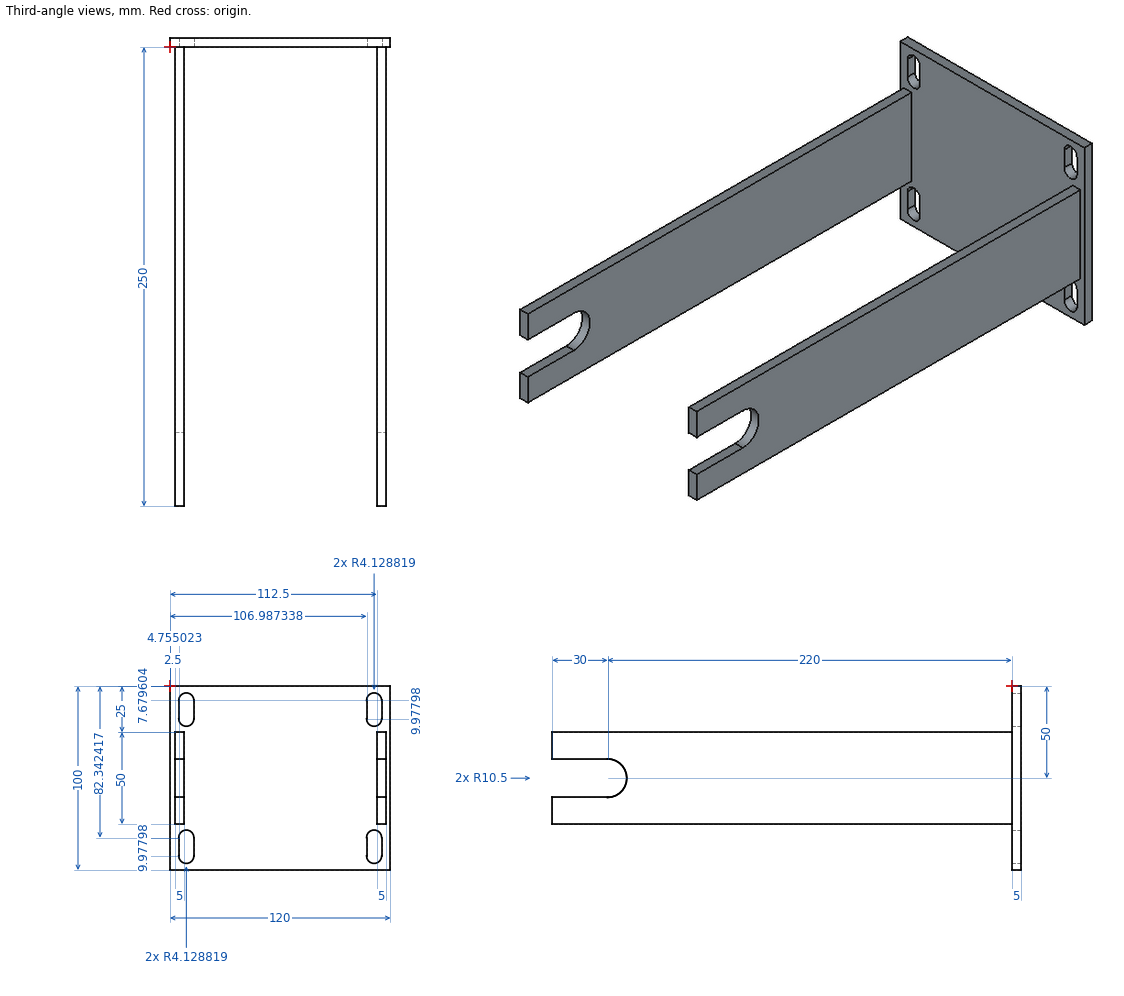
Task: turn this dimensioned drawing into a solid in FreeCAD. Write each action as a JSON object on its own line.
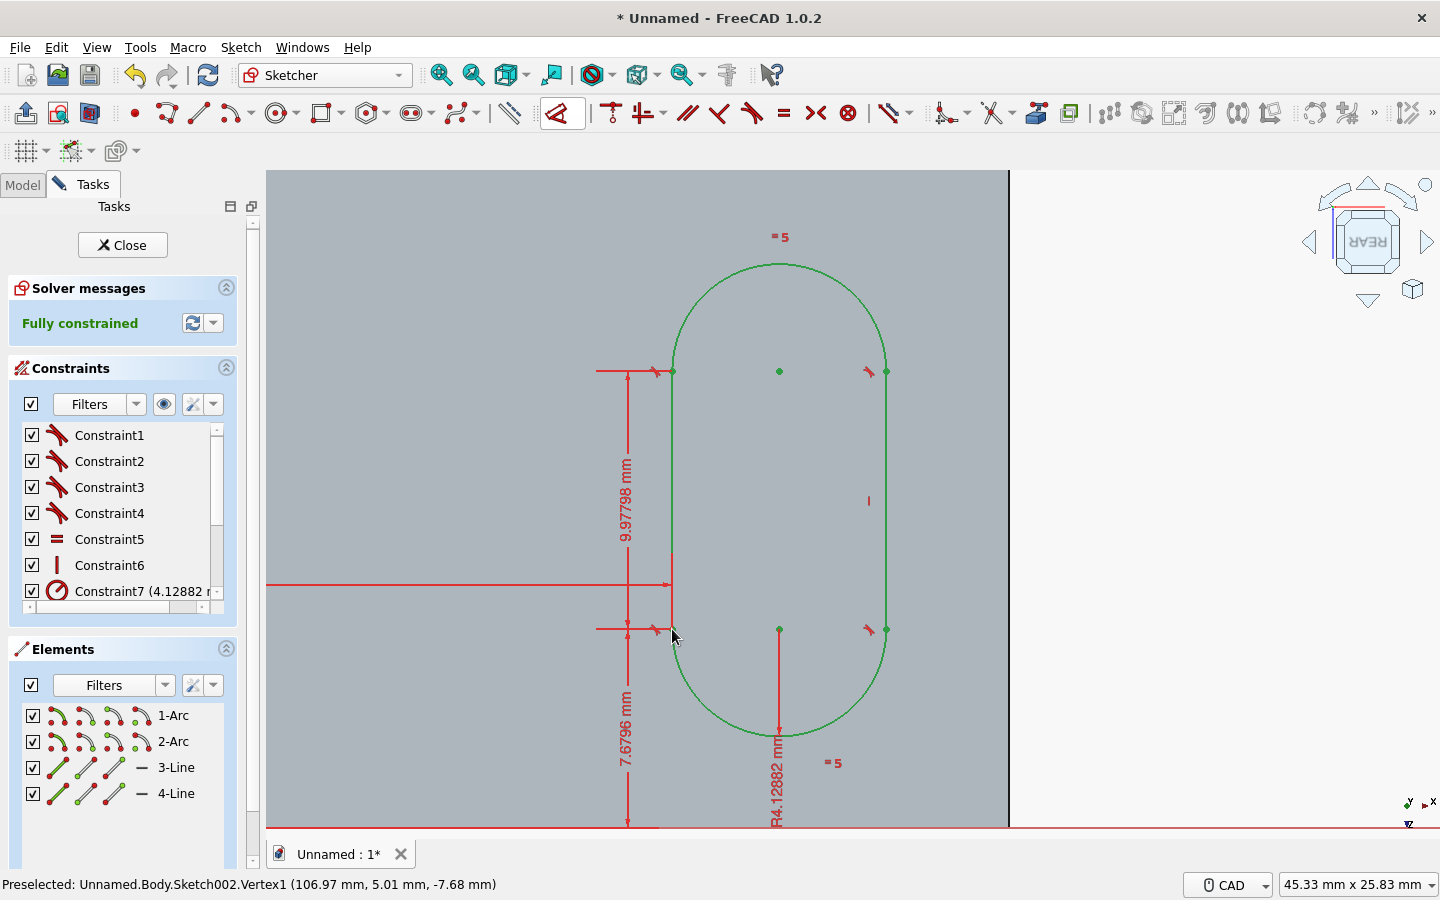
{"action": "left_click", "coordinate": [123, 245]}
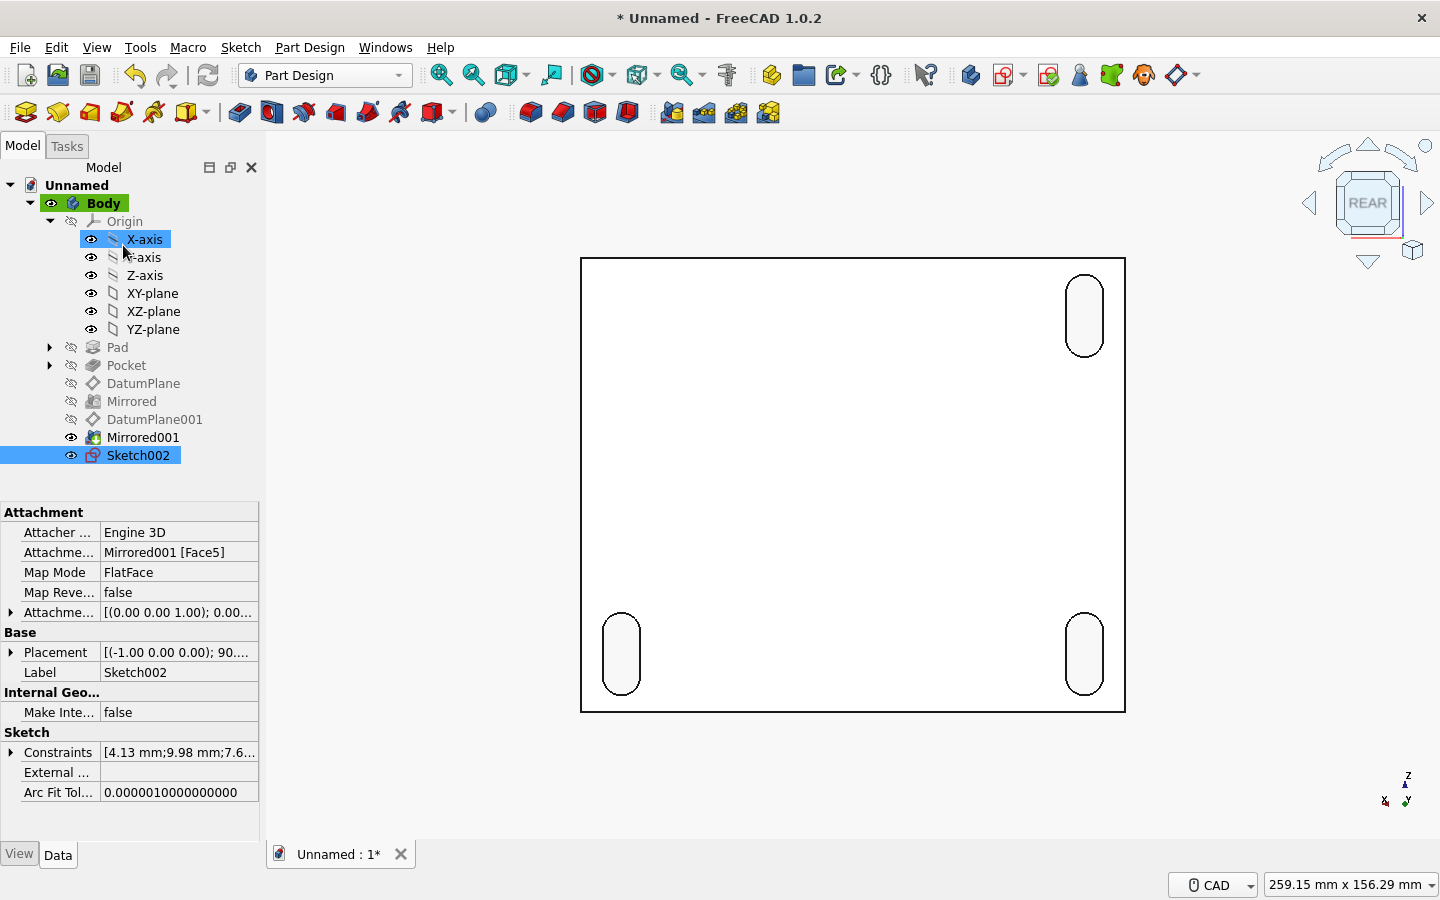
{"action": "left_click", "coordinate": [240, 112]}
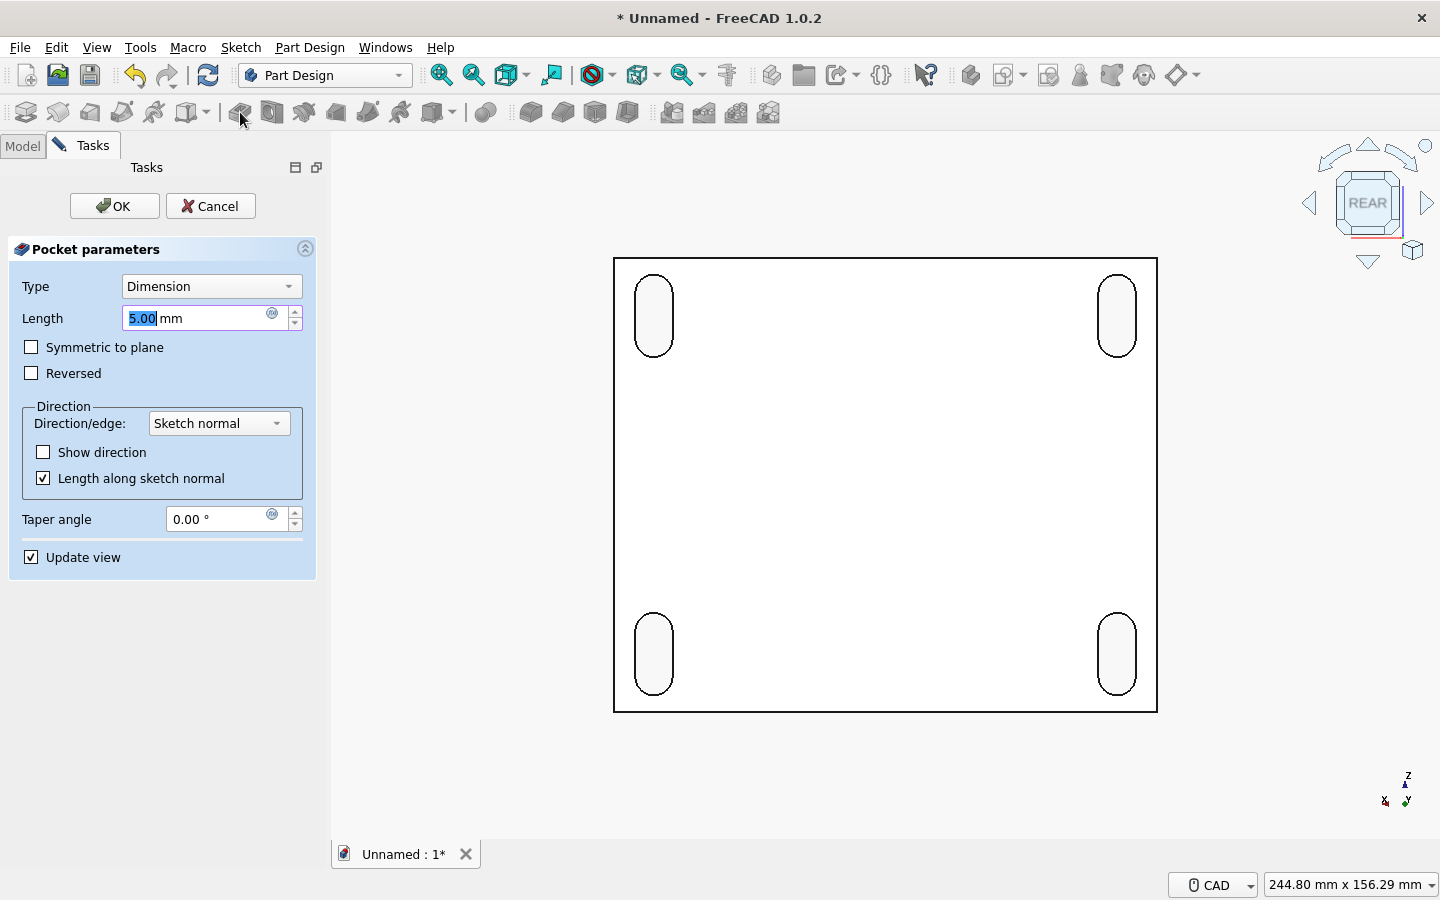
{"action": "left_click", "coordinate": [212, 286]}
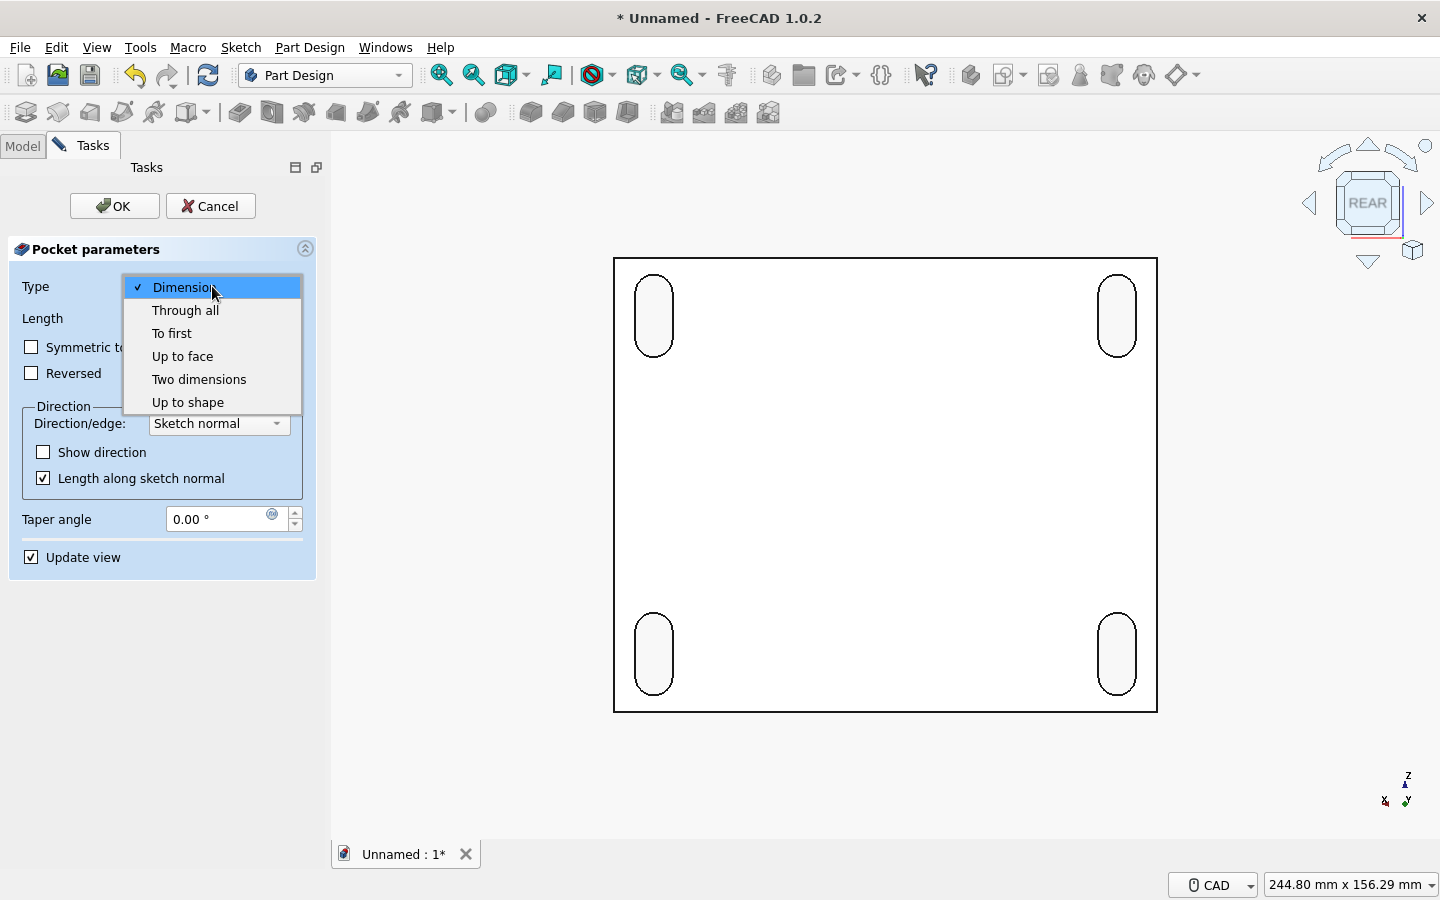
{"action": "left_click", "coordinate": [212, 310]}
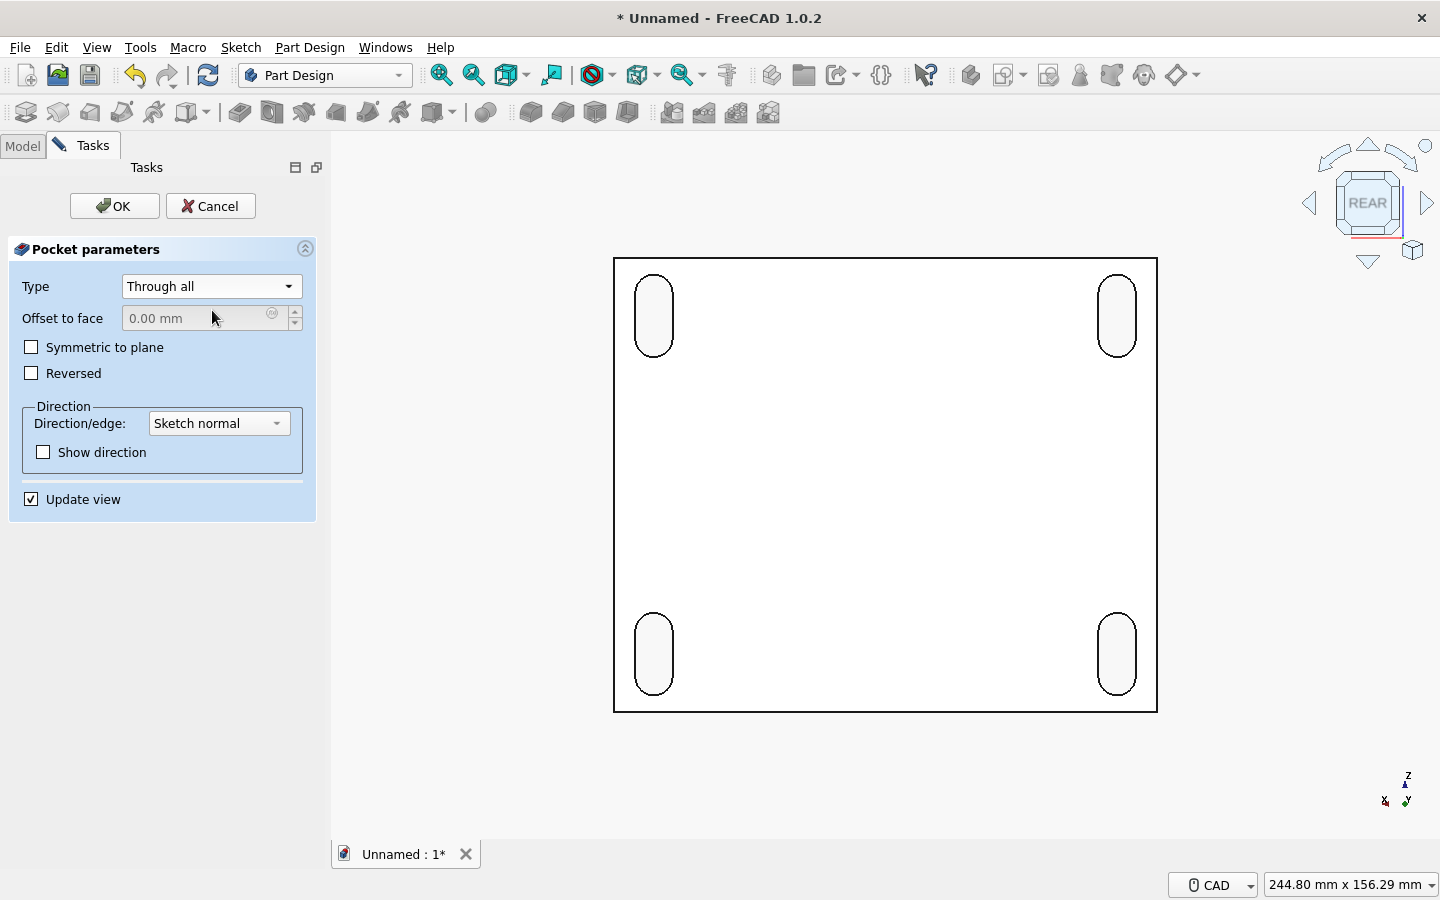
{"action": "left_click", "coordinate": [115, 206]}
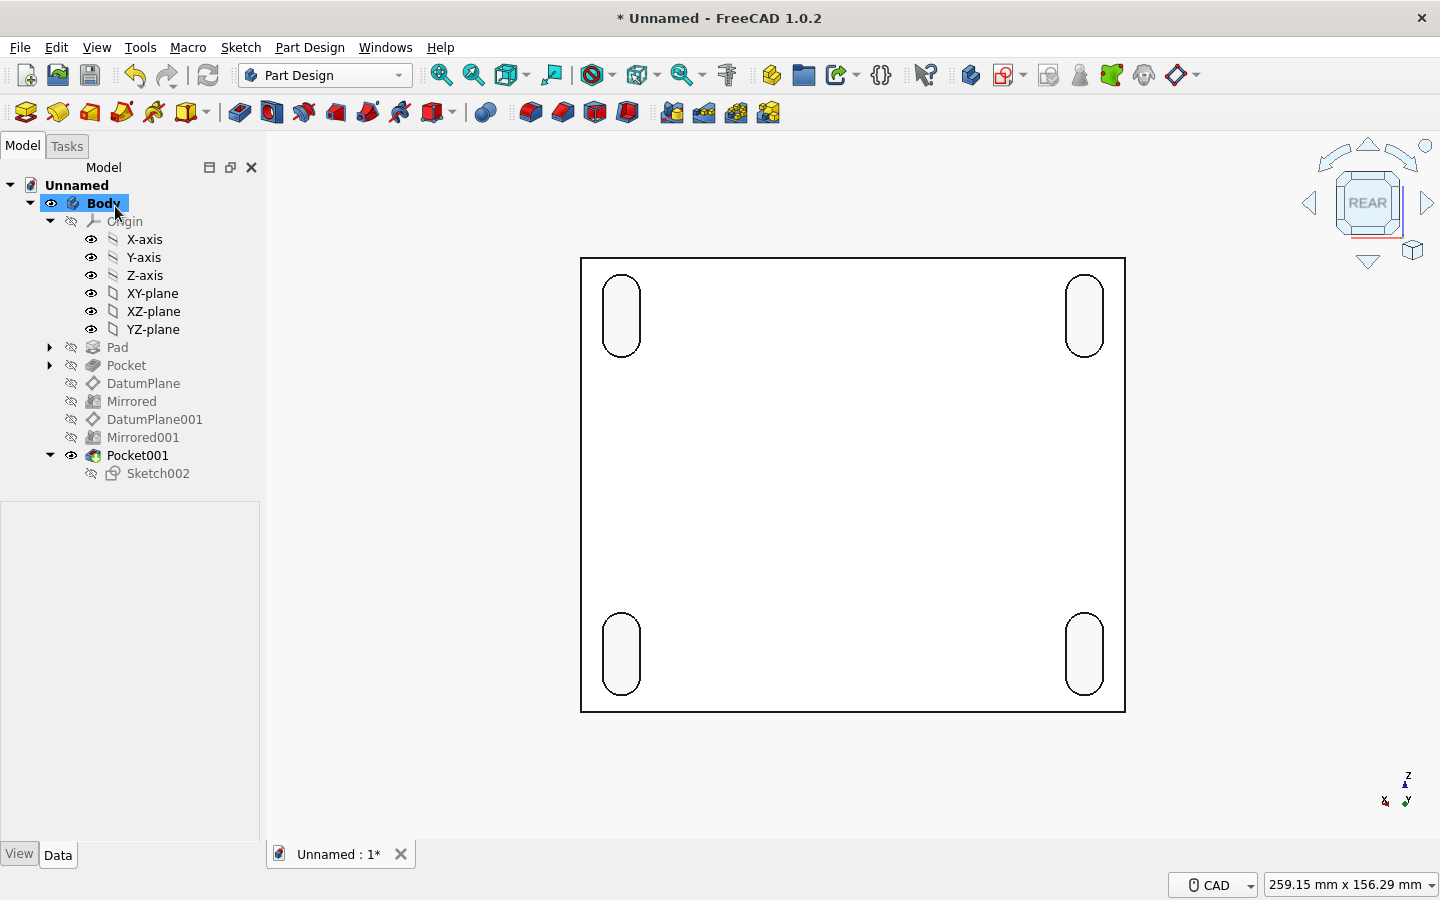
{"action": "left_click", "coordinate": [1004, 76]}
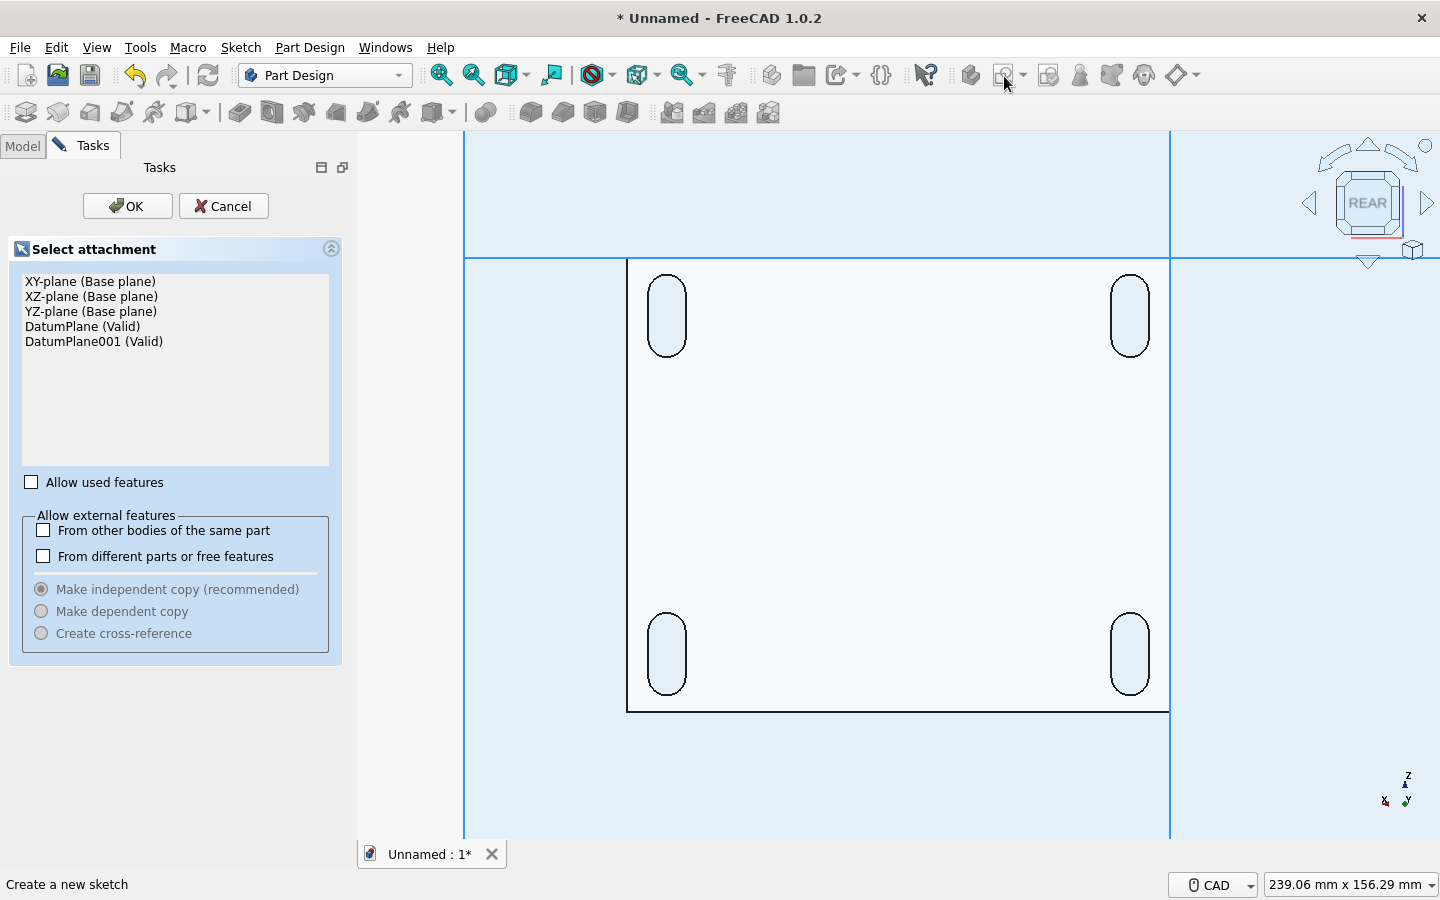
{"action": "left_click", "coordinate": [82, 296]}